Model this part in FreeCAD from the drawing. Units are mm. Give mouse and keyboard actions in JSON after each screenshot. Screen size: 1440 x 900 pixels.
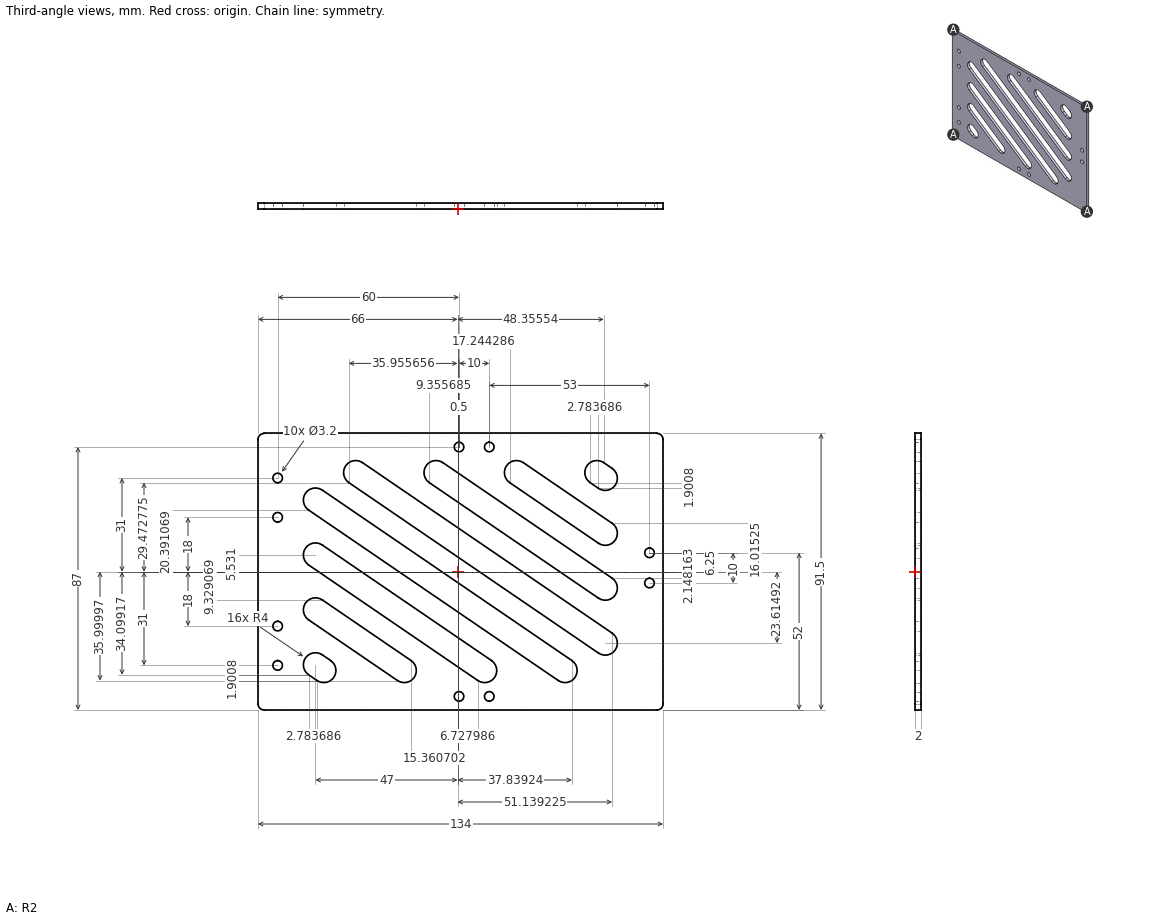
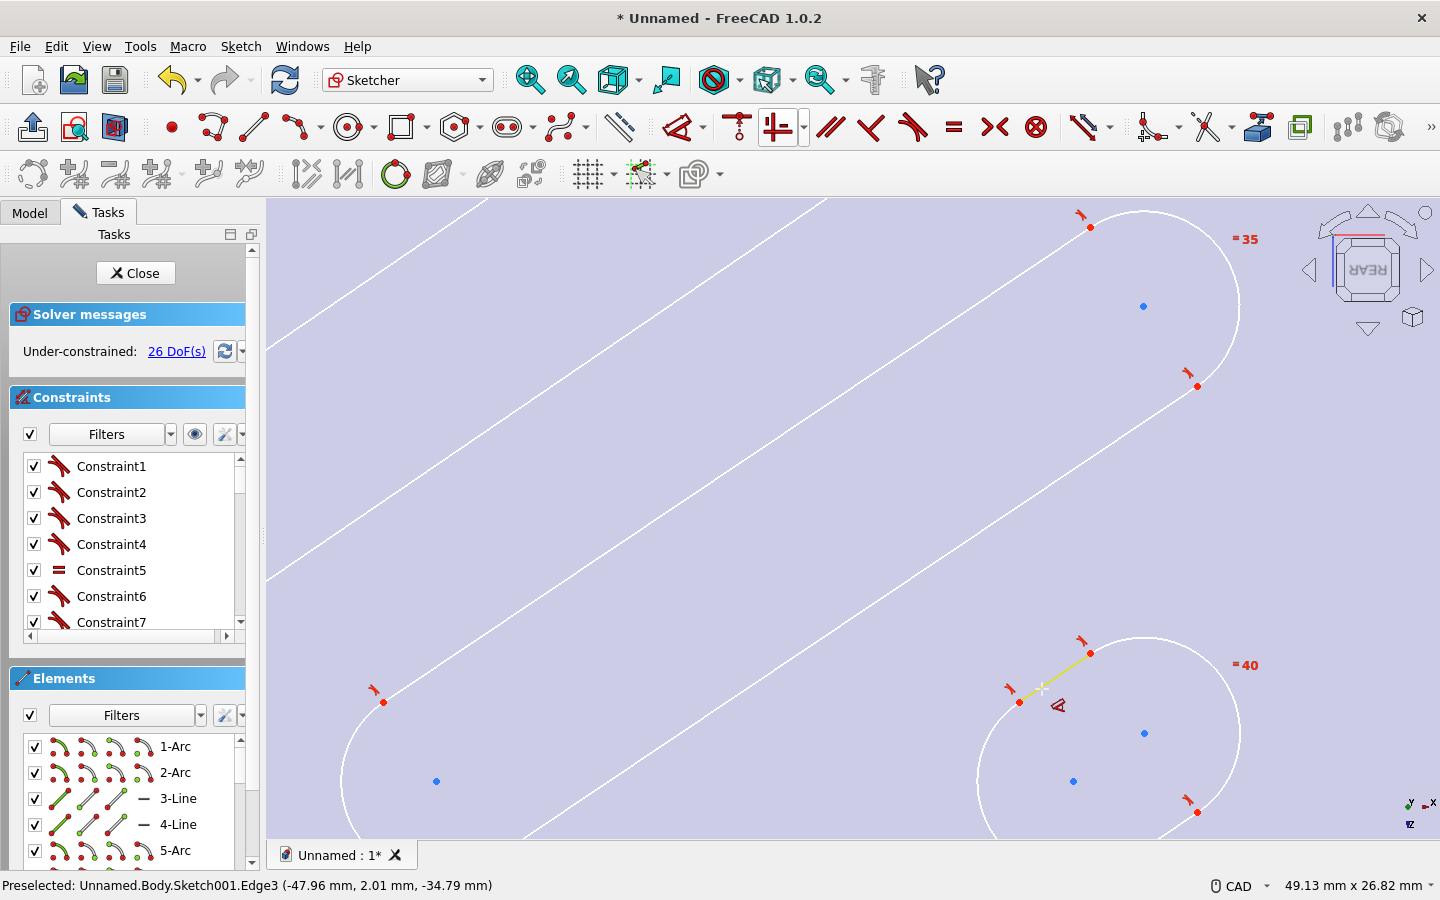
{"action": "left_click", "coordinate": [1041, 688]}
{"action": "left_click", "coordinate": [1125, 678]}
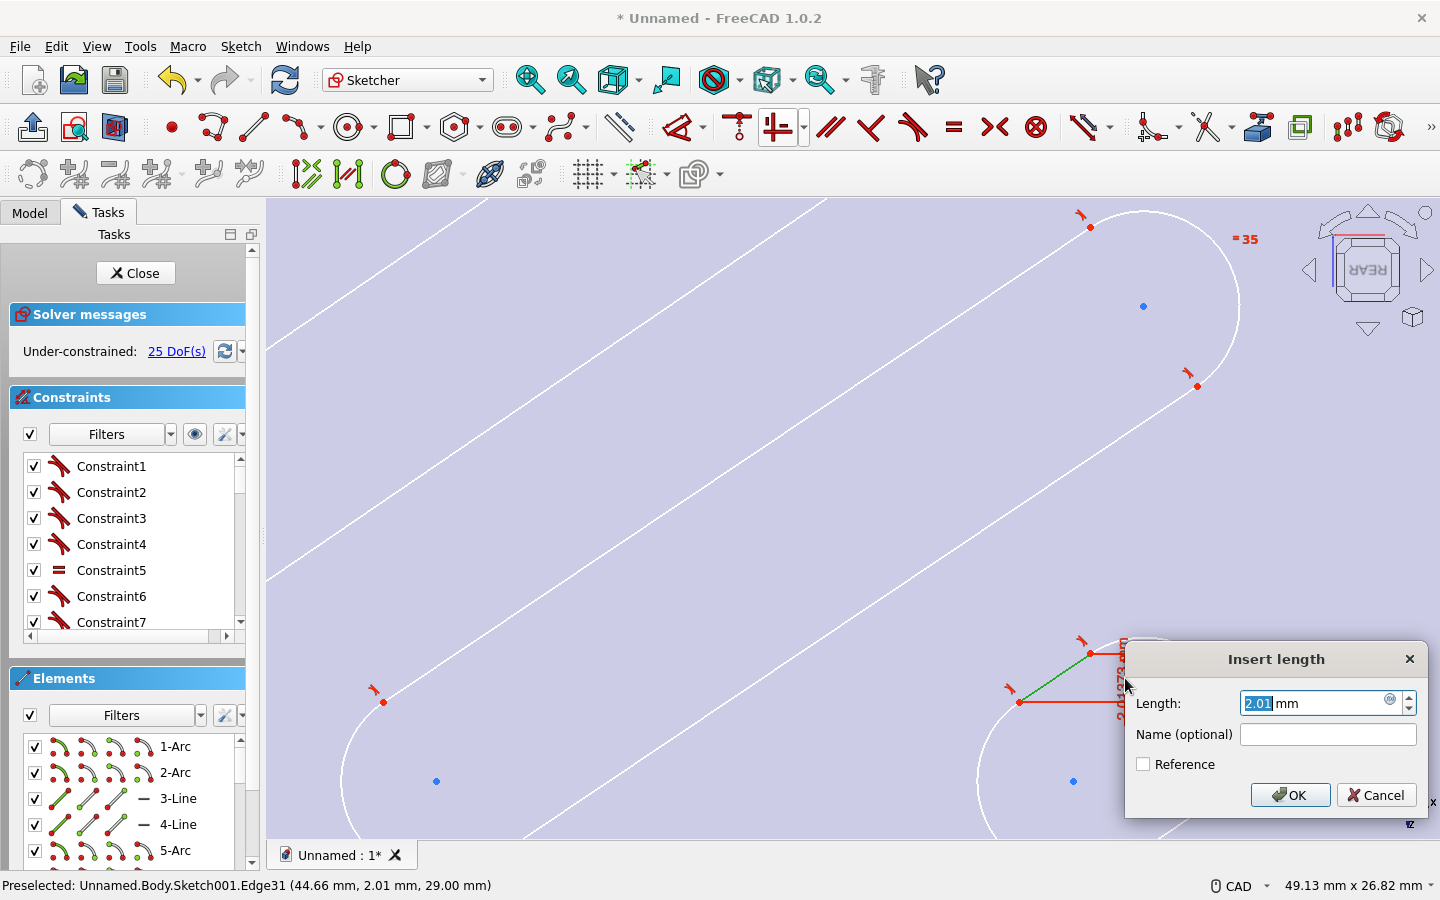
{"action": "type", "text": "1.9008"}
{"action": "key", "text": "Return"}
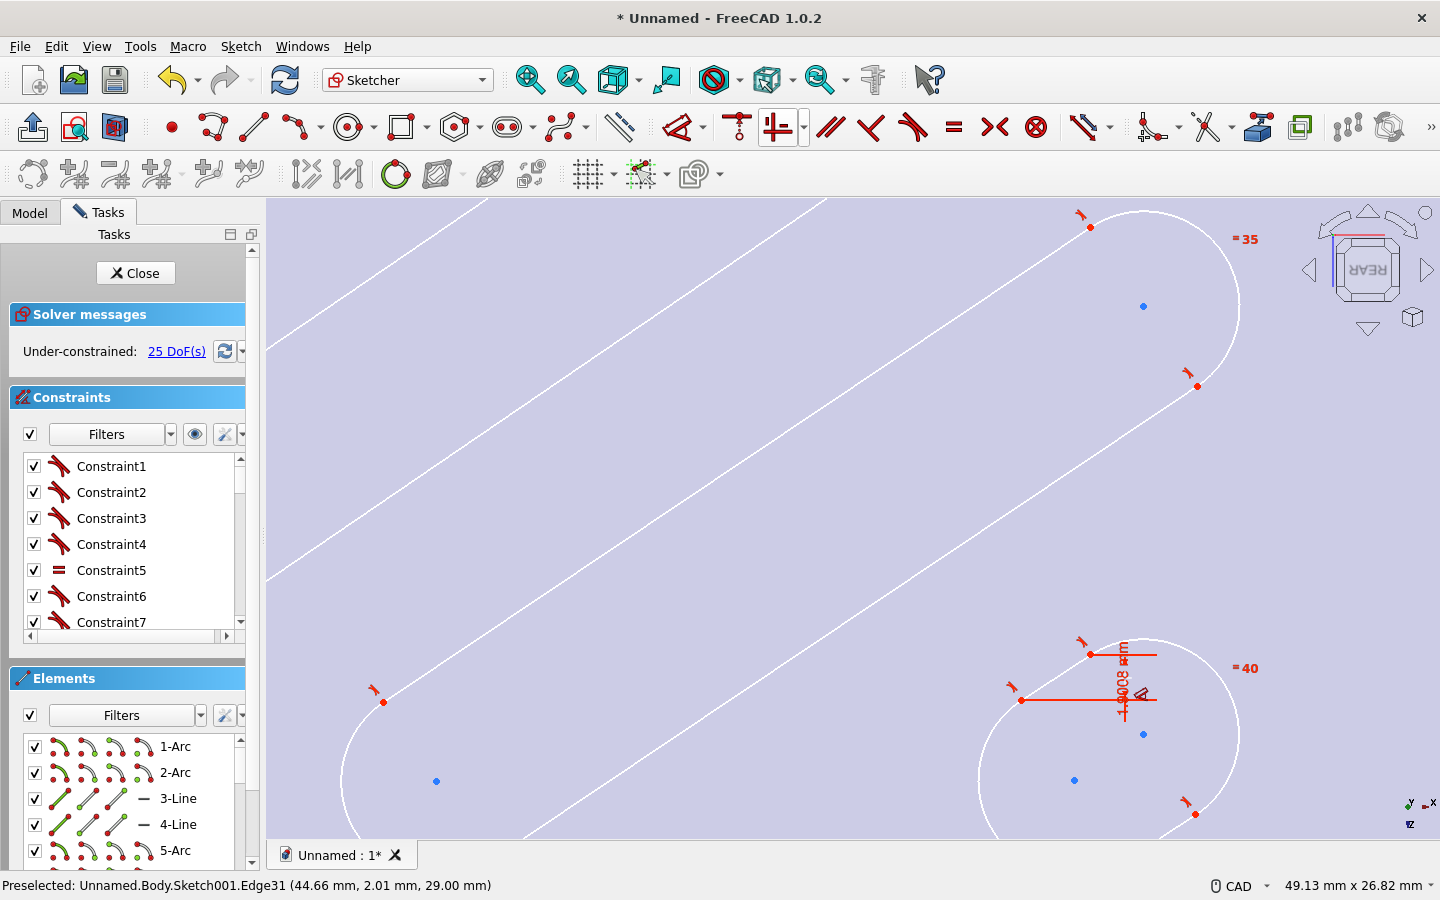
{"action": "scroll", "coordinate": [1043, 690], "scroll_direction": "down", "scroll_amount": 7}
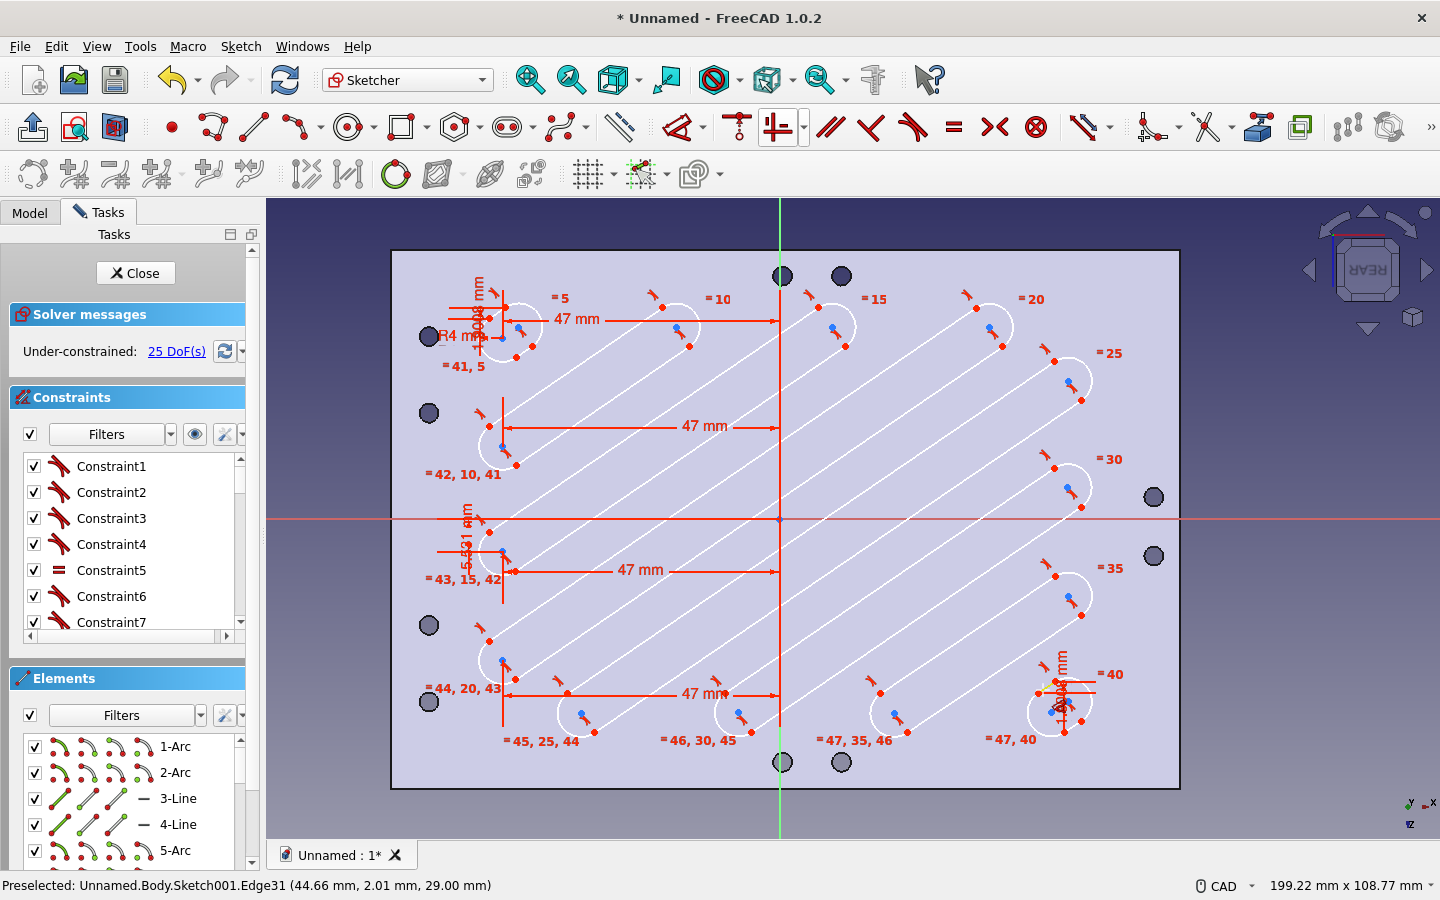
{"action": "left_click", "coordinate": [489, 319]}
{"action": "left_click", "coordinate": [455, 419]}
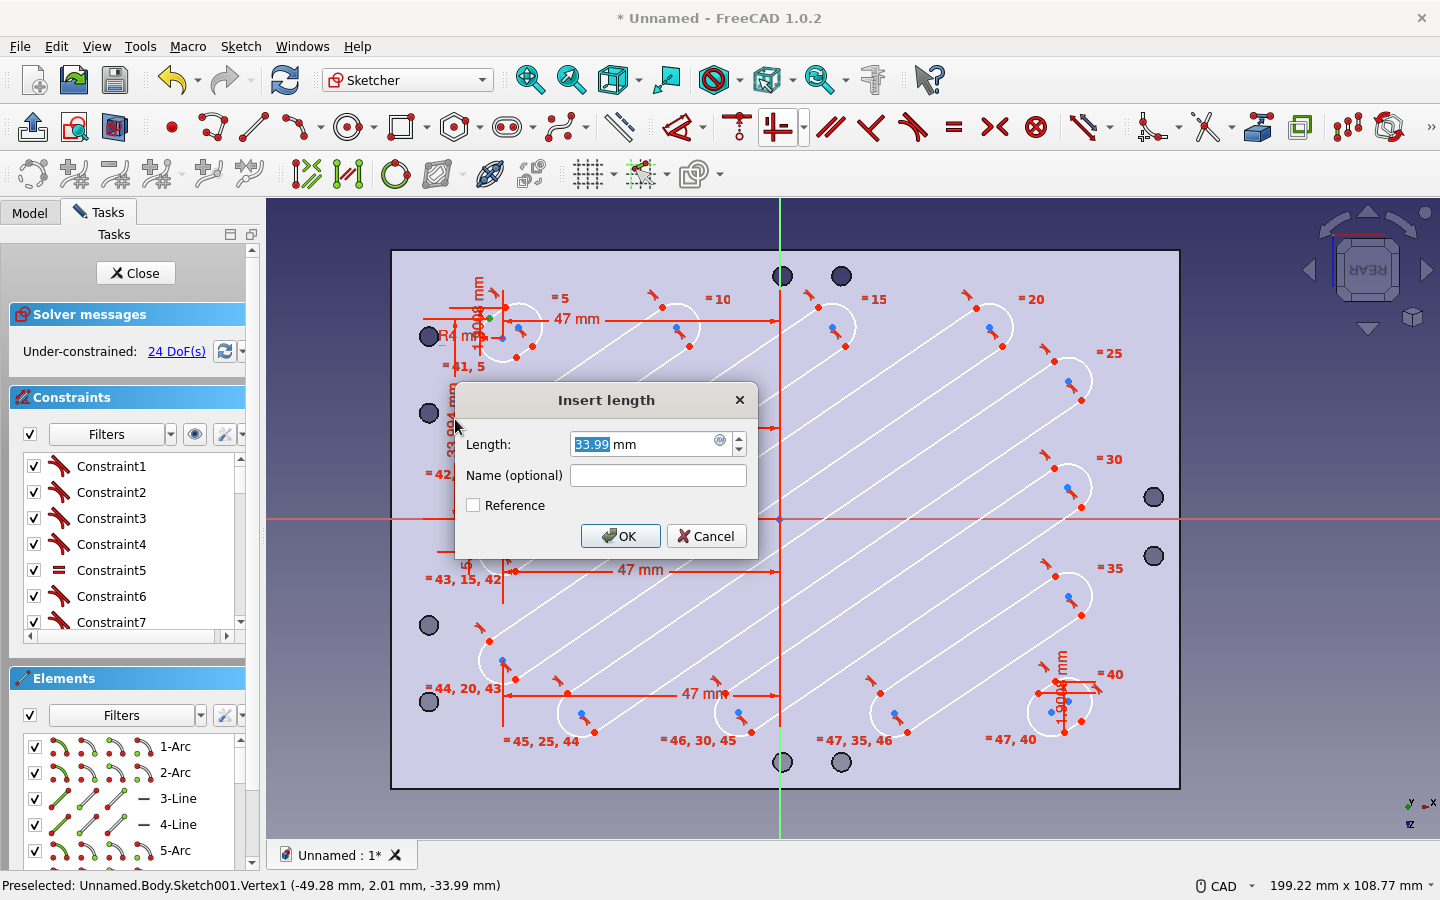
{"action": "type", "text": "34.09917"}
{"action": "key", "text": "Return"}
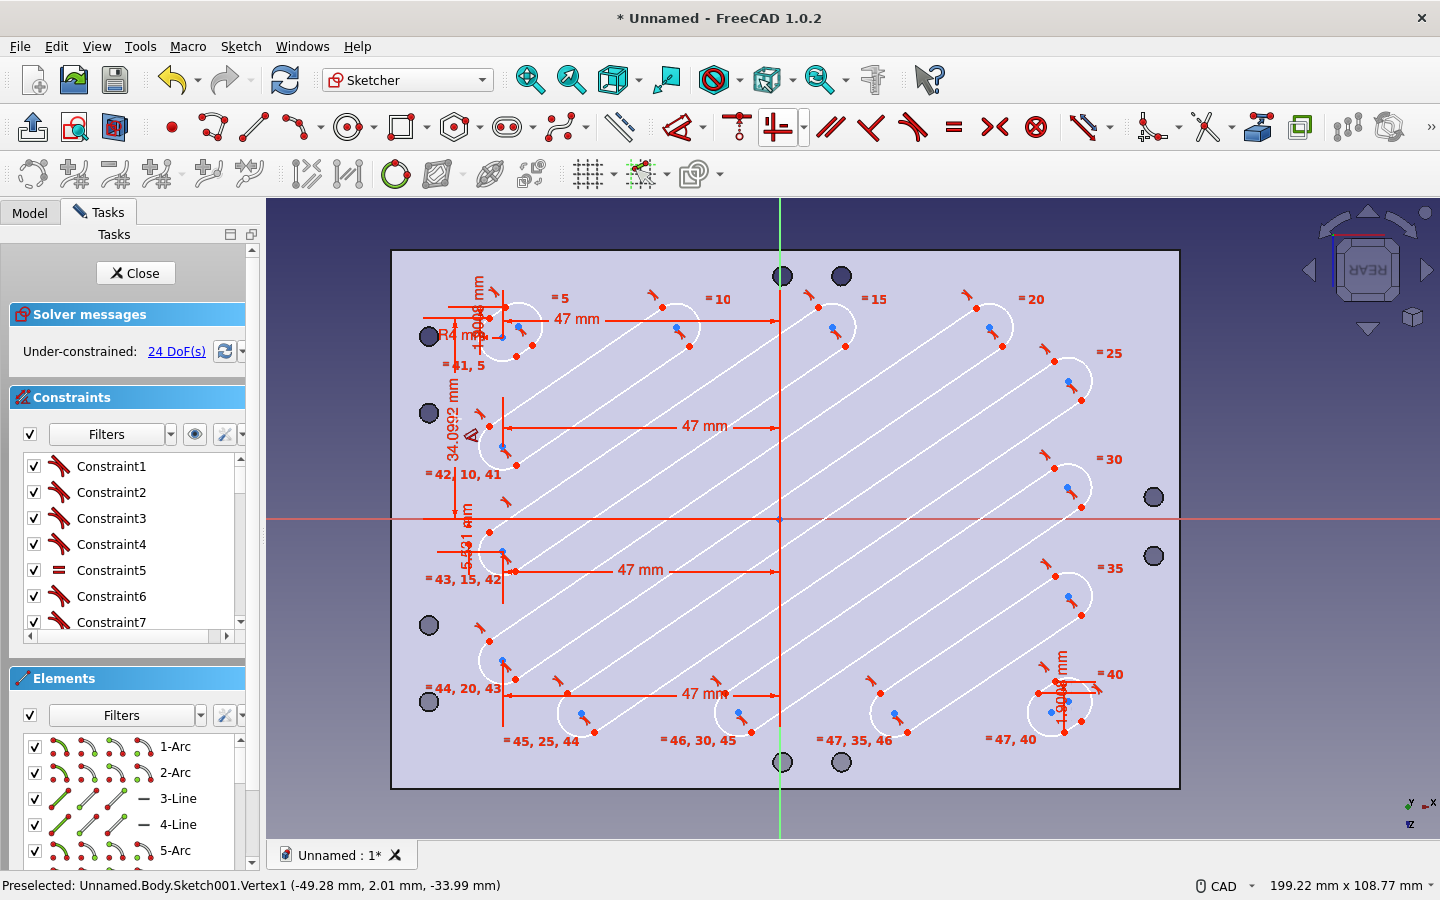
{"action": "left_click", "coordinate": [516, 466]}
{"action": "left_click", "coordinate": [482, 492]}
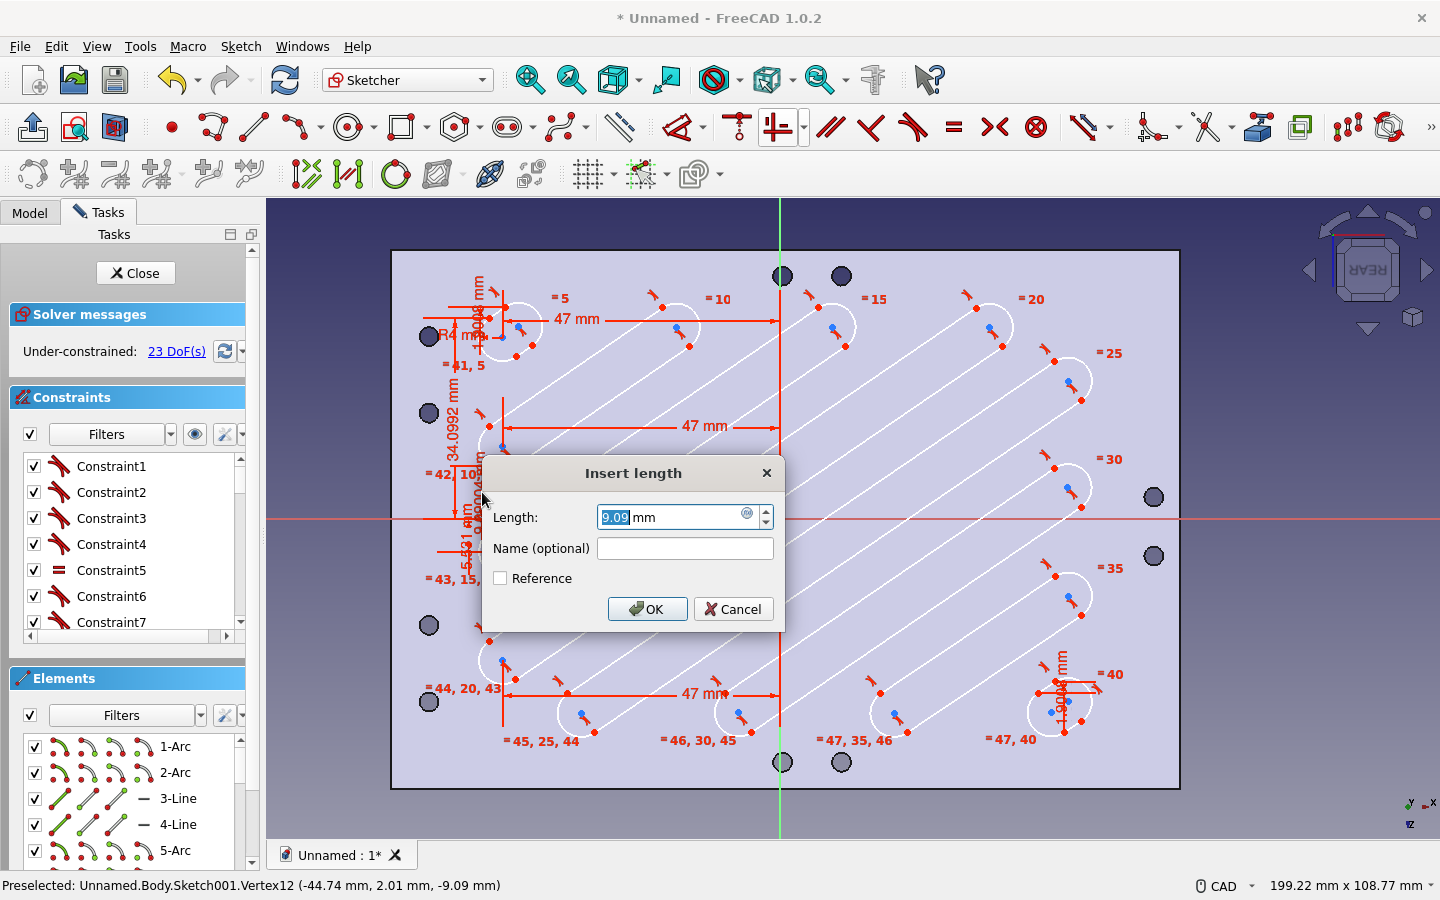
{"action": "type", "text": "9.329069"}
{"action": "key", "text": "Return"}